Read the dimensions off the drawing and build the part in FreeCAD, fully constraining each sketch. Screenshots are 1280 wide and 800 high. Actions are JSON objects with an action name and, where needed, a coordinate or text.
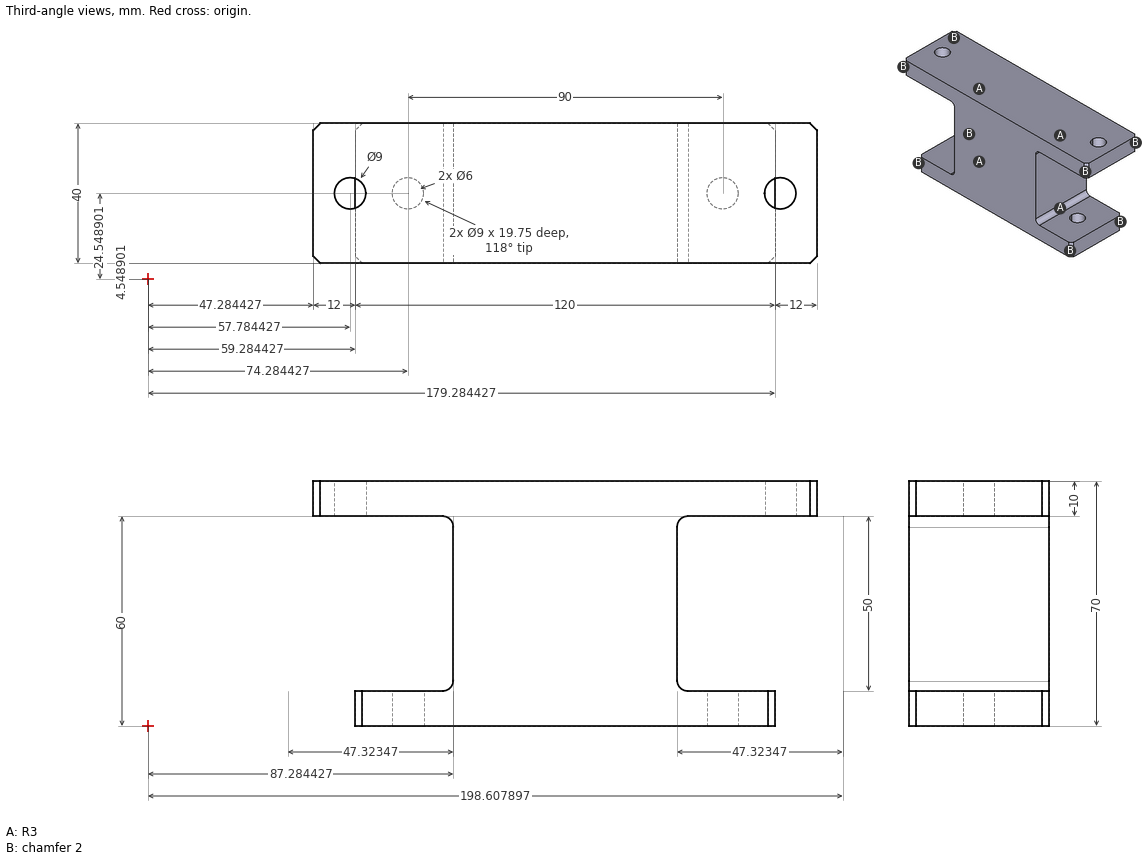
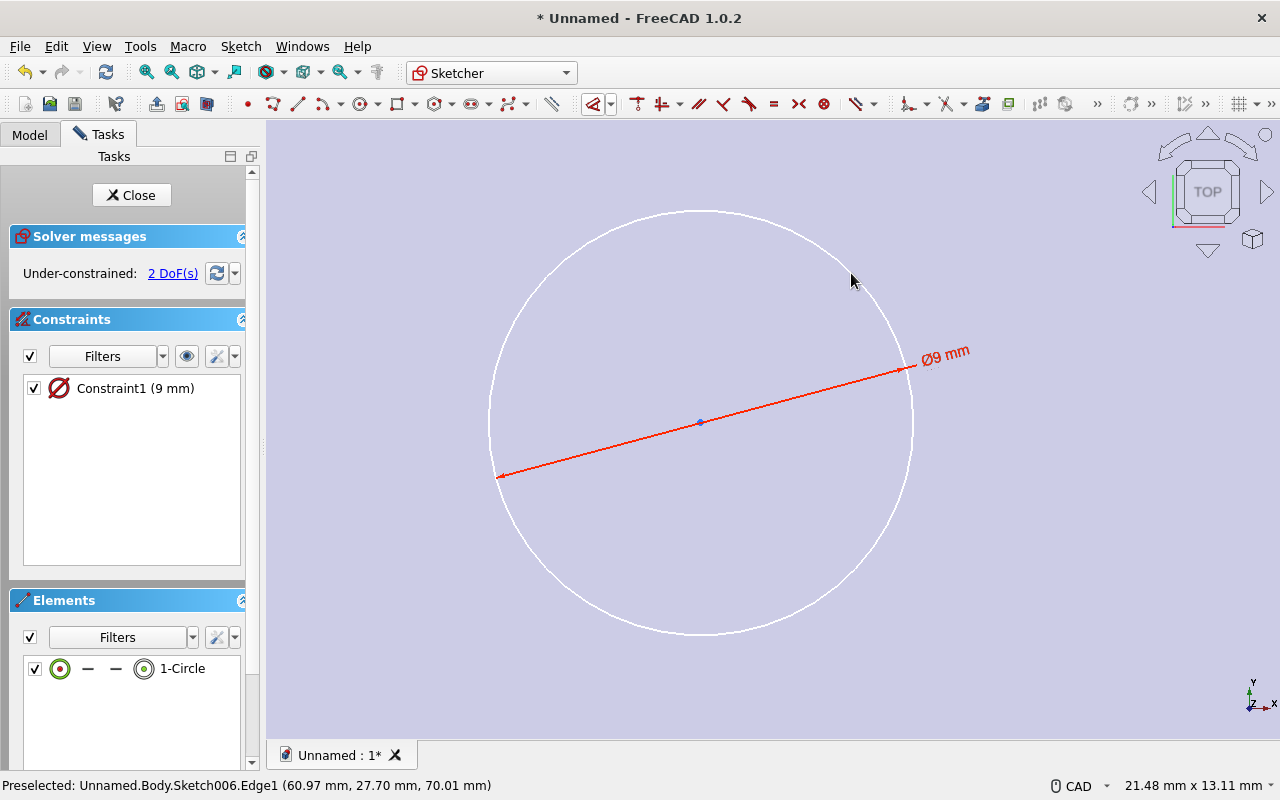
{"action": "left_click", "coordinate": [701, 423]}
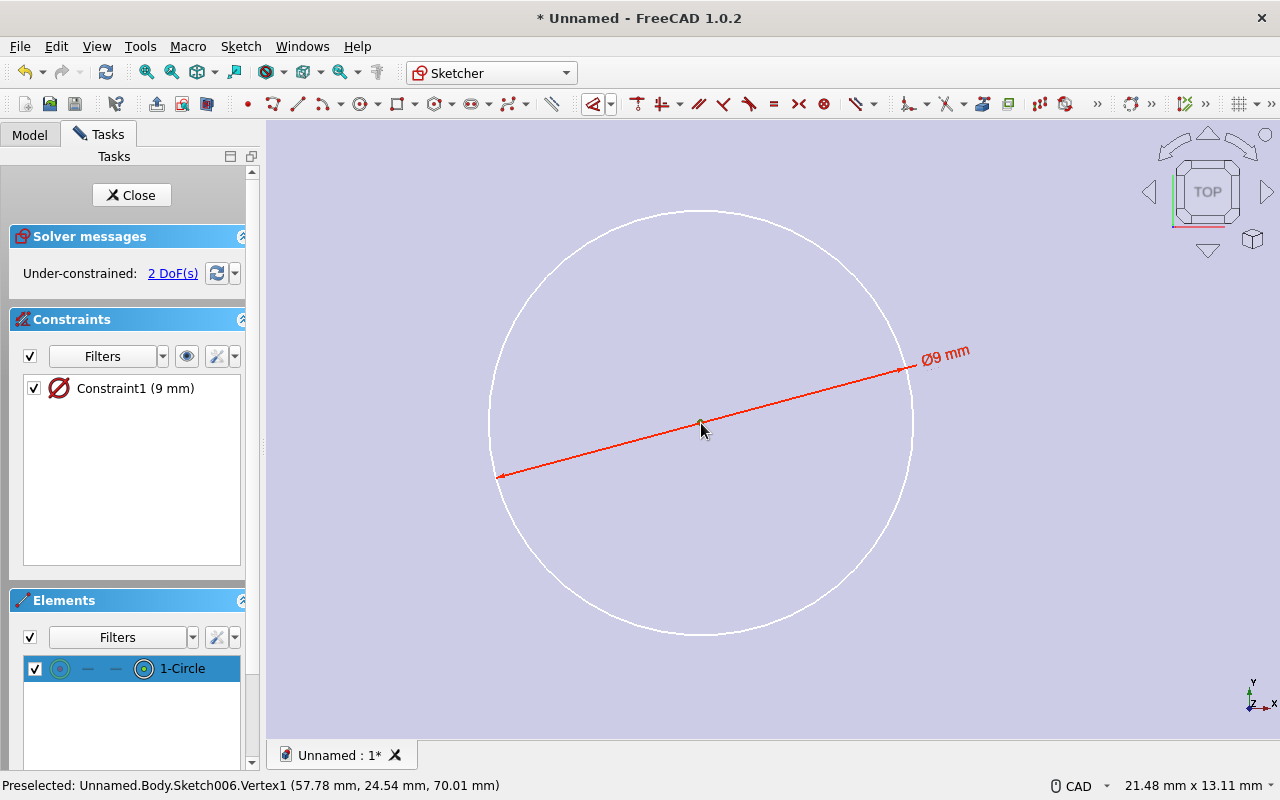
{"action": "key", "text": "l"}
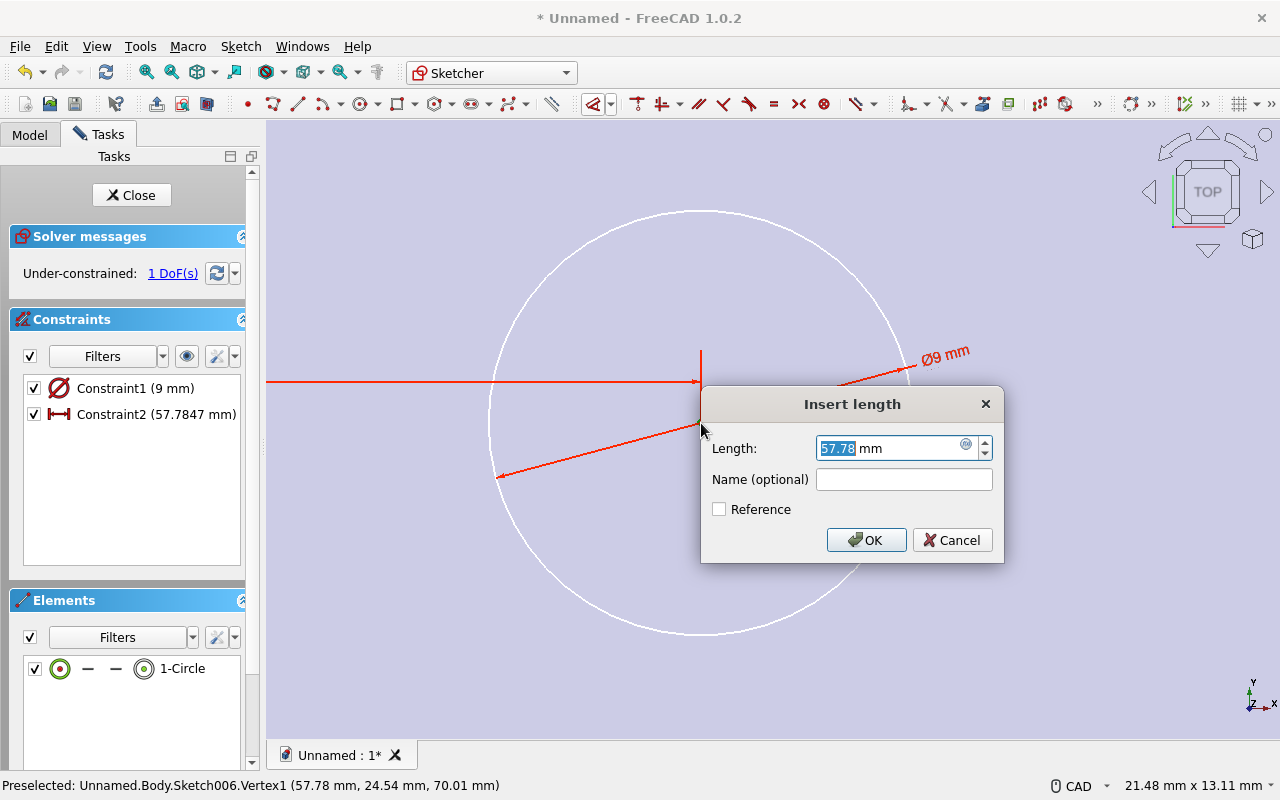
{"action": "type", "text": "57.784427"}
{"action": "key", "text": "Return"}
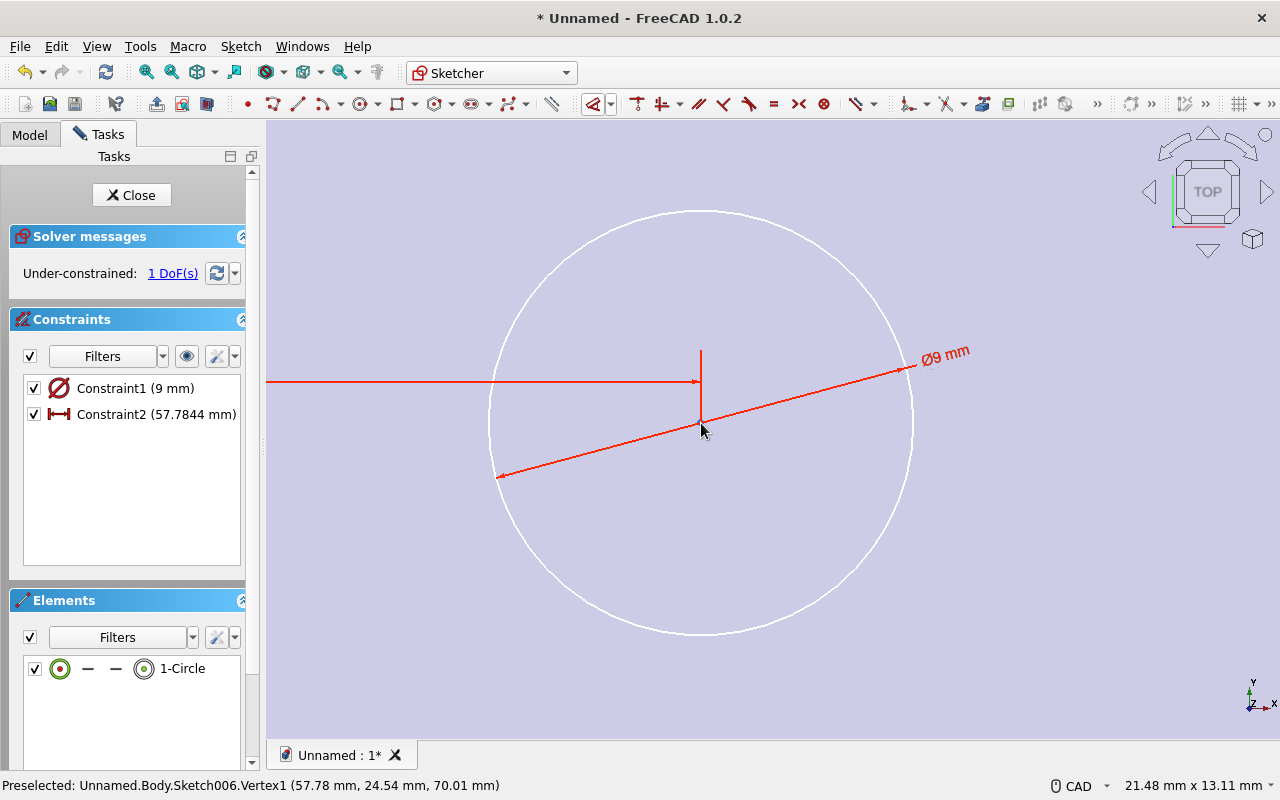
{"action": "left_click", "coordinate": [701, 423]}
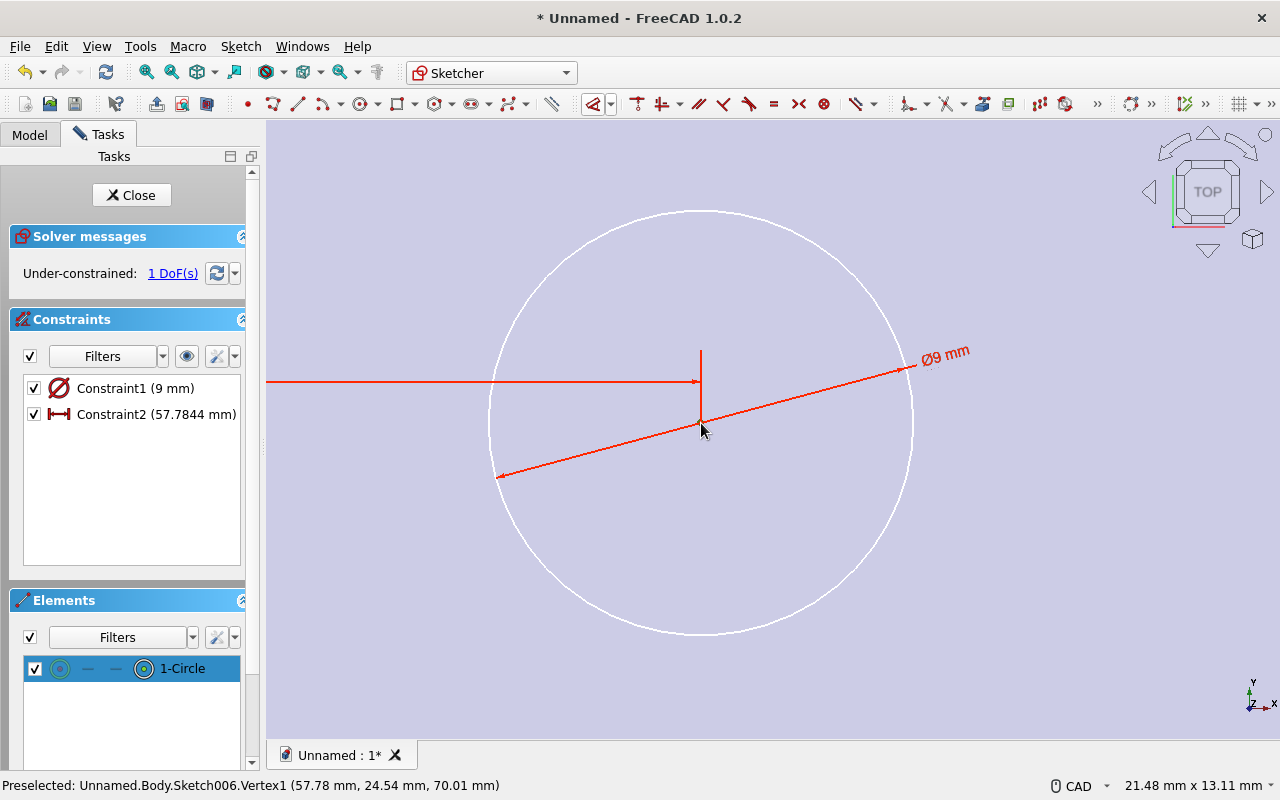
{"action": "key", "text": "i"}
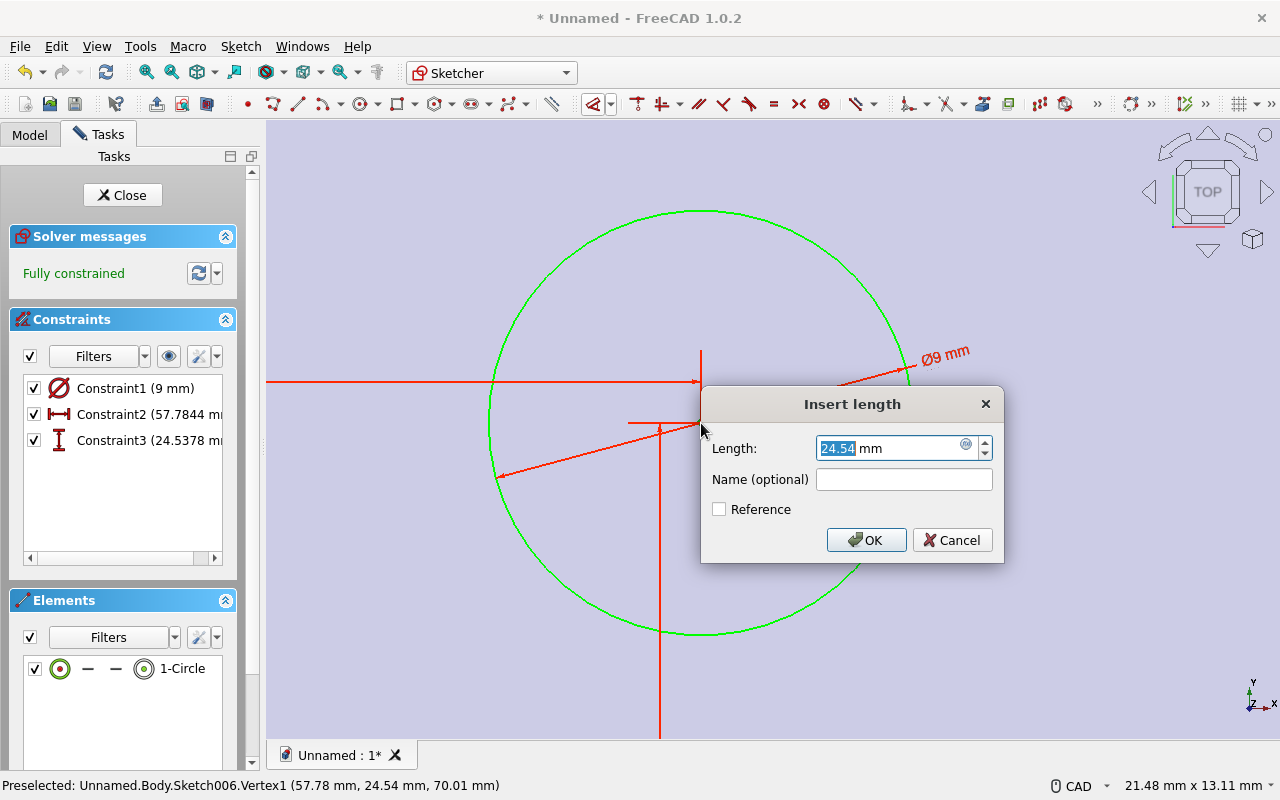
{"action": "type", "text": "24.548901"}
{"action": "key", "text": "Return"}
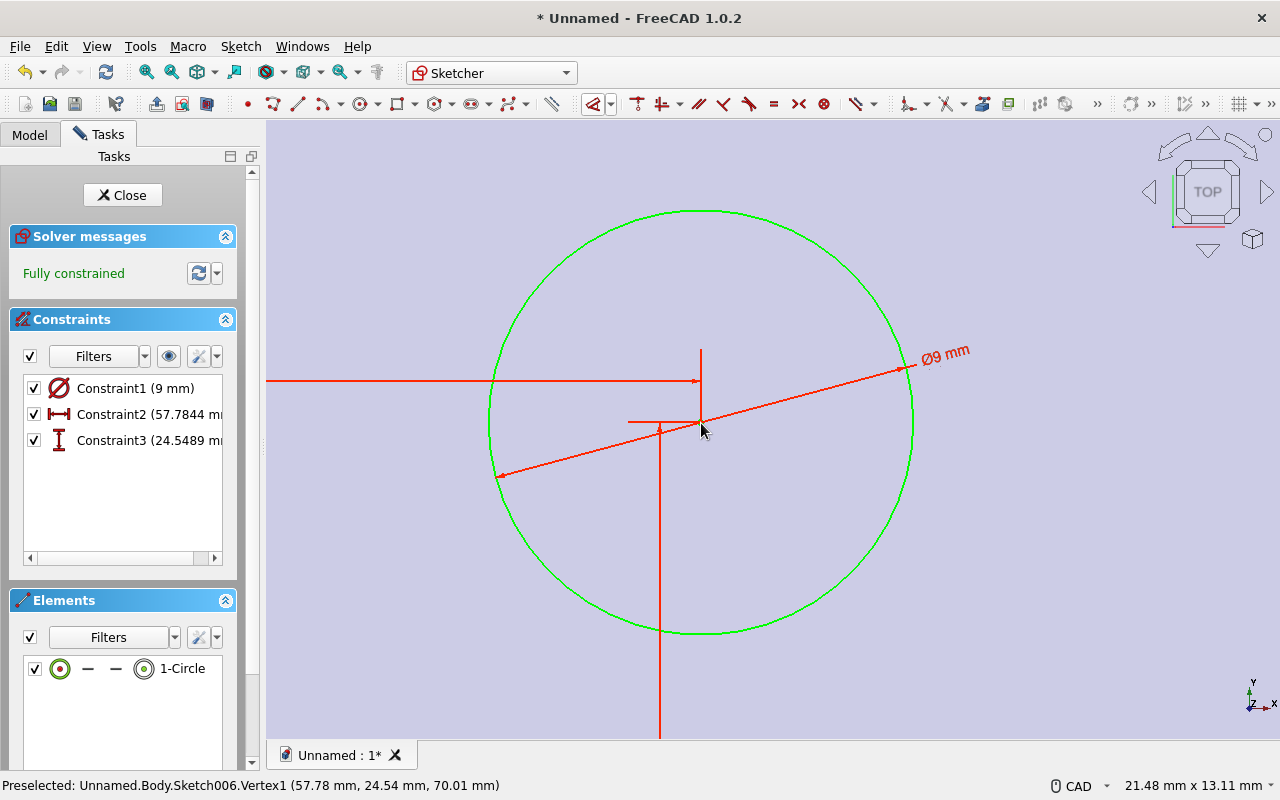
{"action": "left_click", "coordinate": [123, 195]}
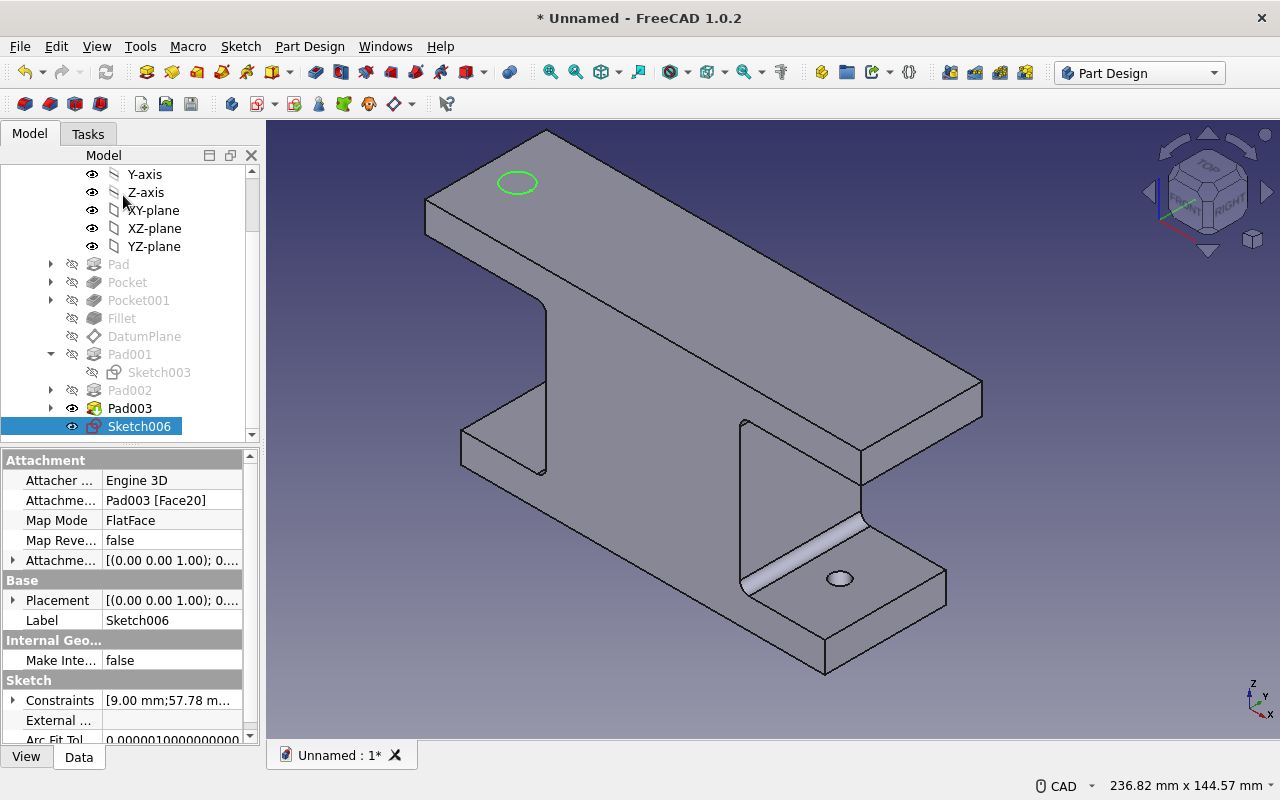
{"action": "left_click", "coordinate": [316, 72]}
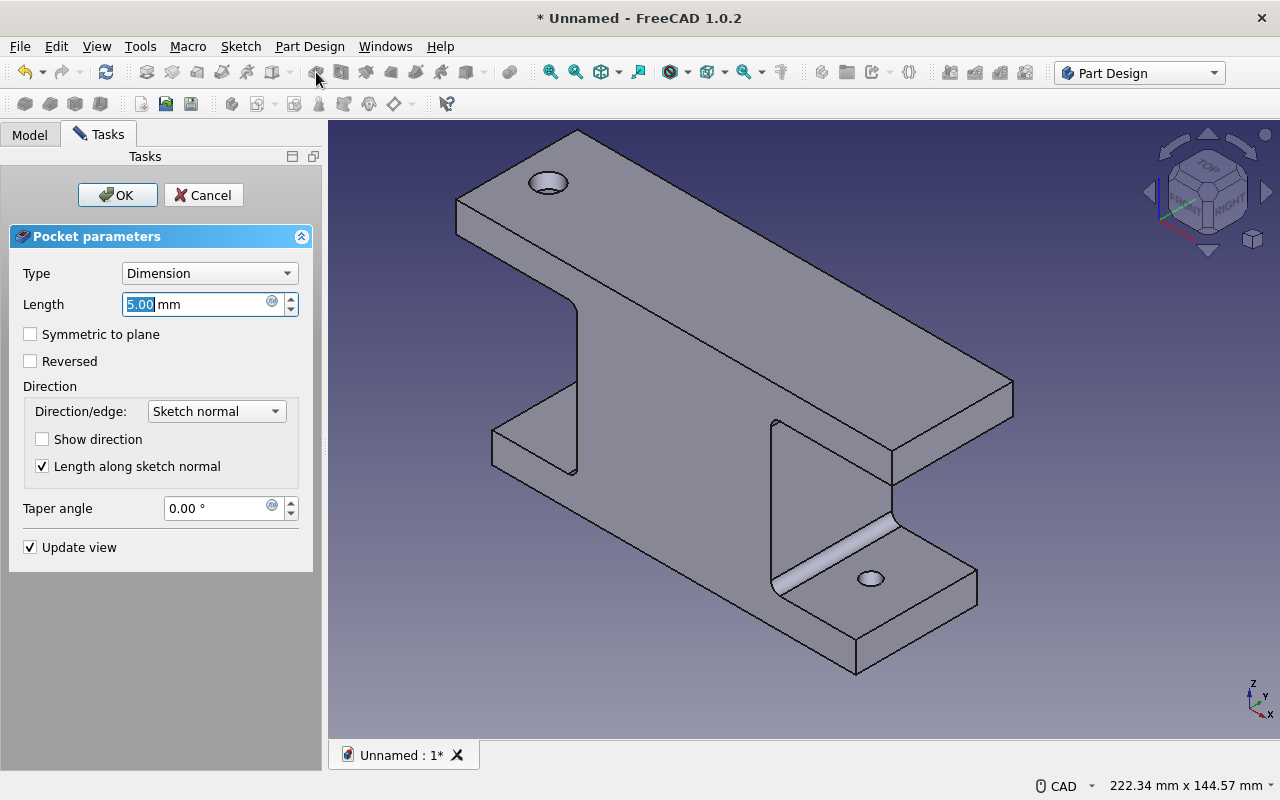
{"action": "type", "text": "10"}
{"action": "key", "text": "Tab"}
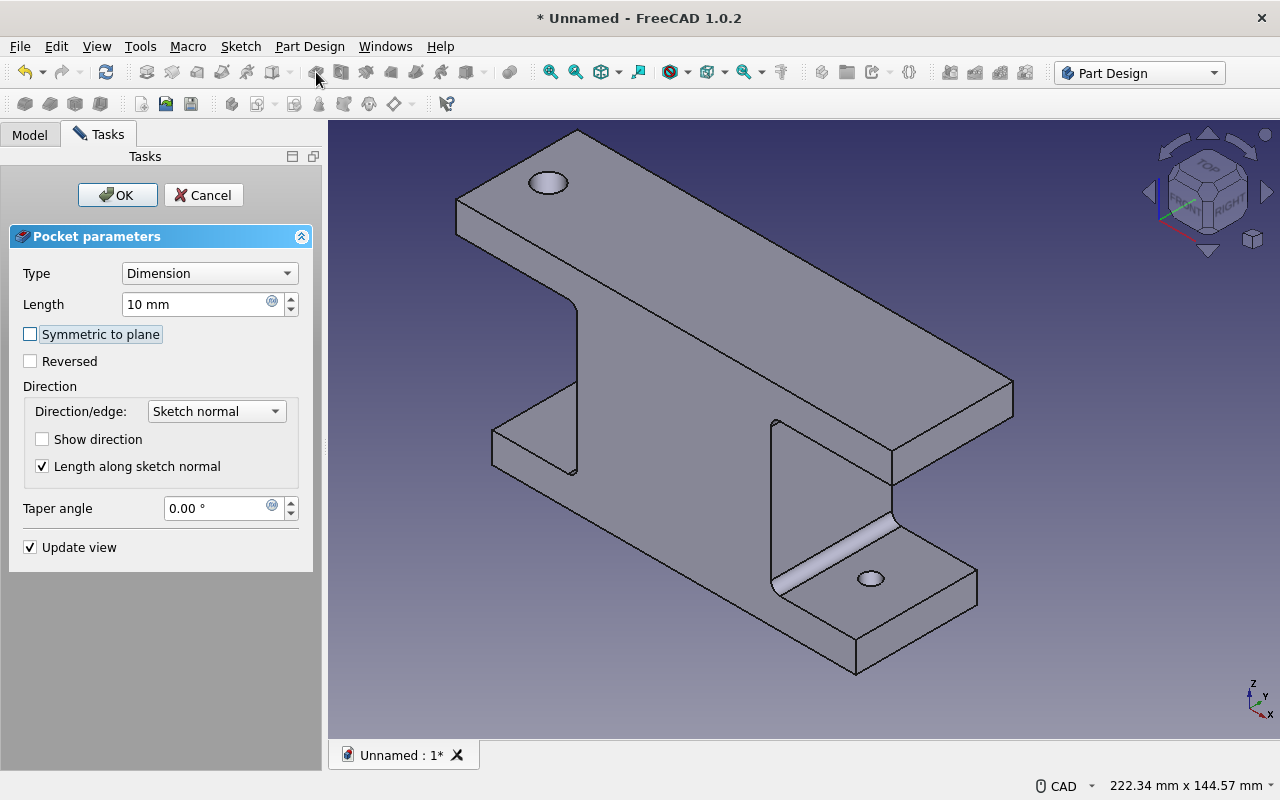
{"action": "left_click", "coordinate": [118, 195]}